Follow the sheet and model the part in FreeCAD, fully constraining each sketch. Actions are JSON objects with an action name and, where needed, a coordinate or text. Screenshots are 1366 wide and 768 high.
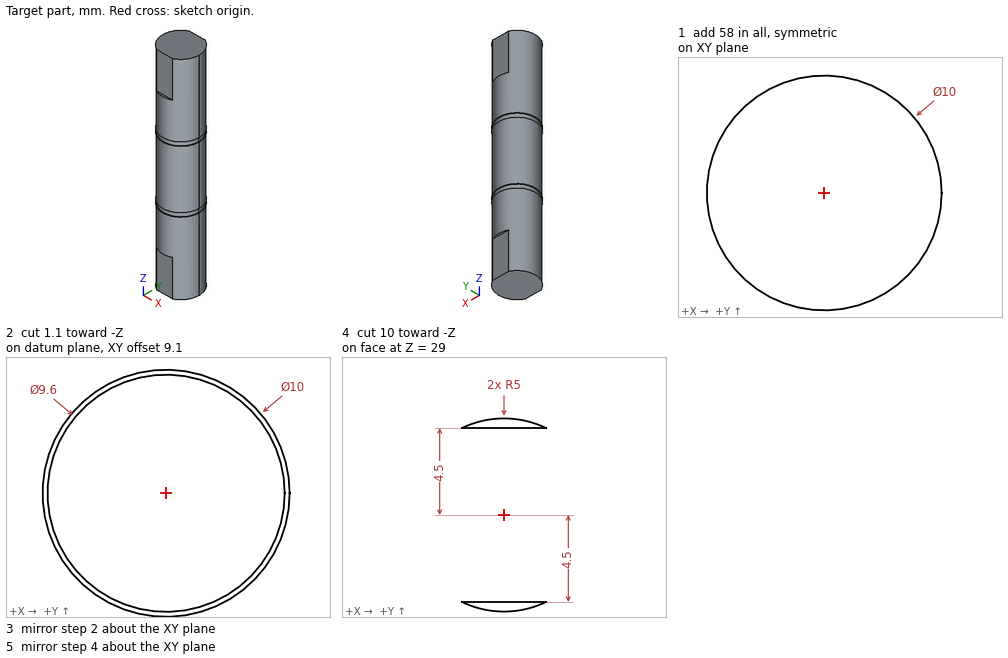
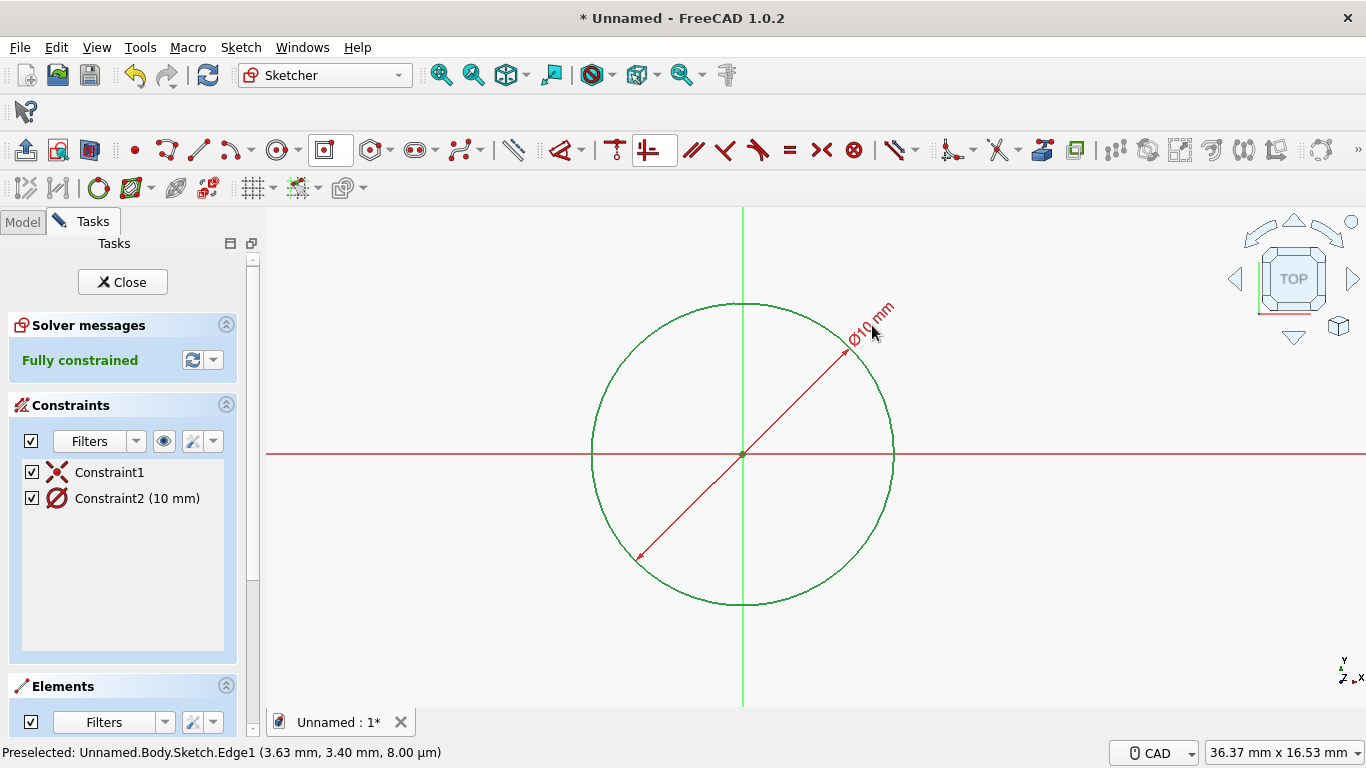
{"action": "left_click", "coordinate": [123, 282]}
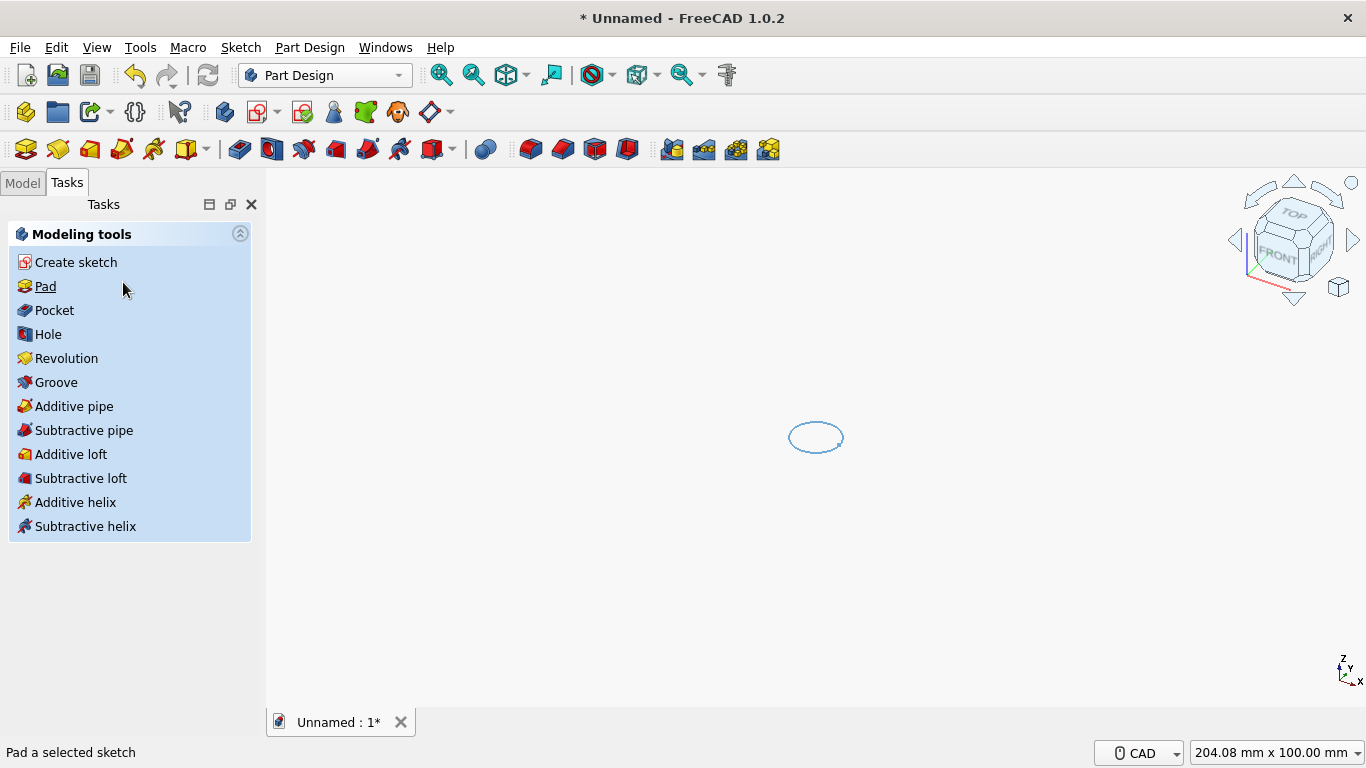
{"action": "left_click", "coordinate": [26, 150]}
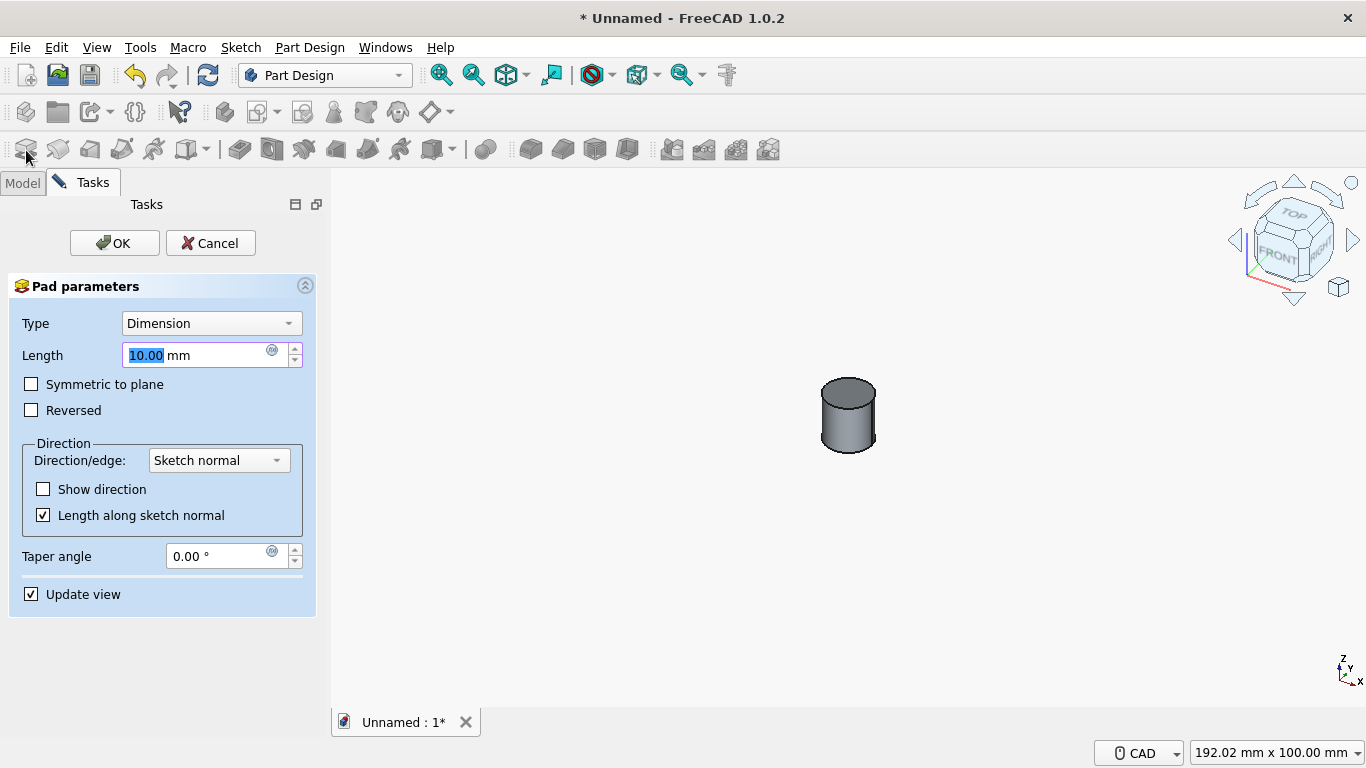
{"action": "type", "text": "58"}
{"action": "key", "text": "Tab"}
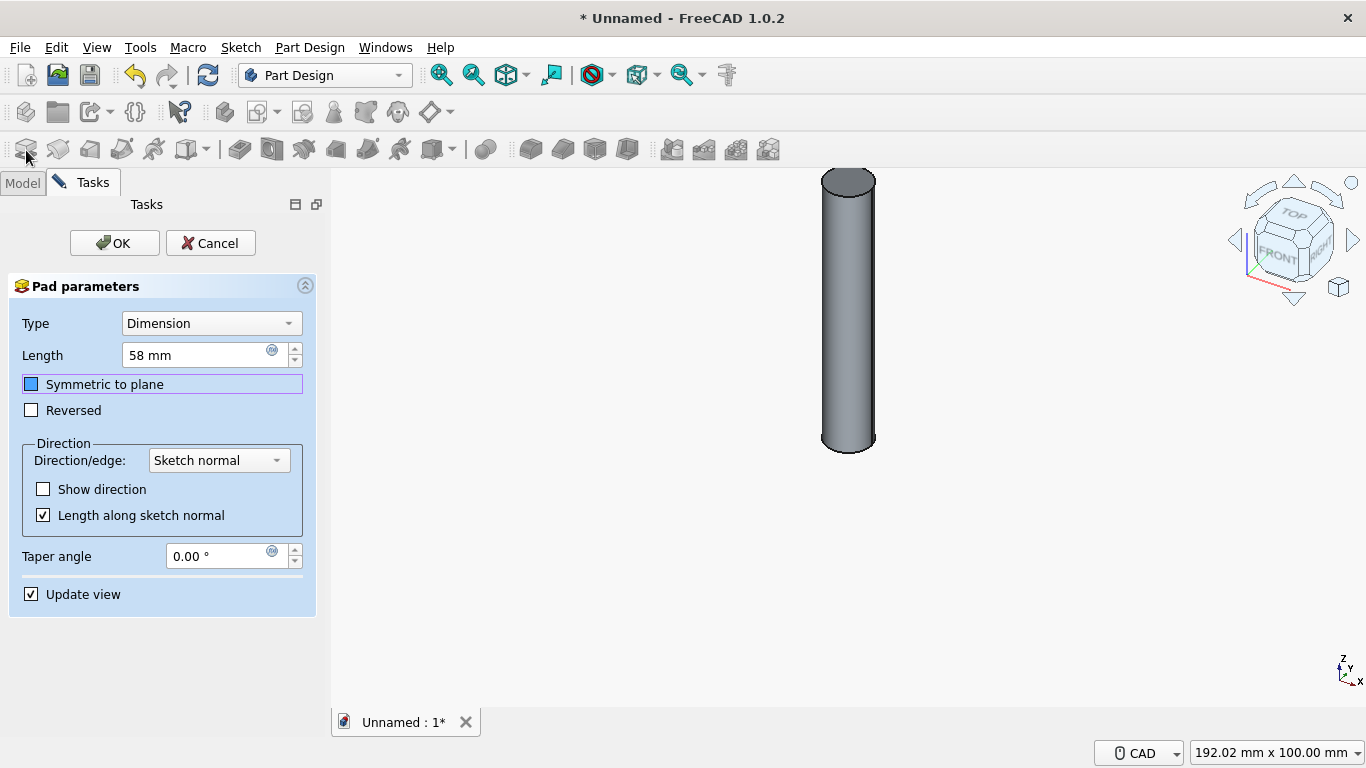
{"action": "left_click", "coordinate": [30, 384]}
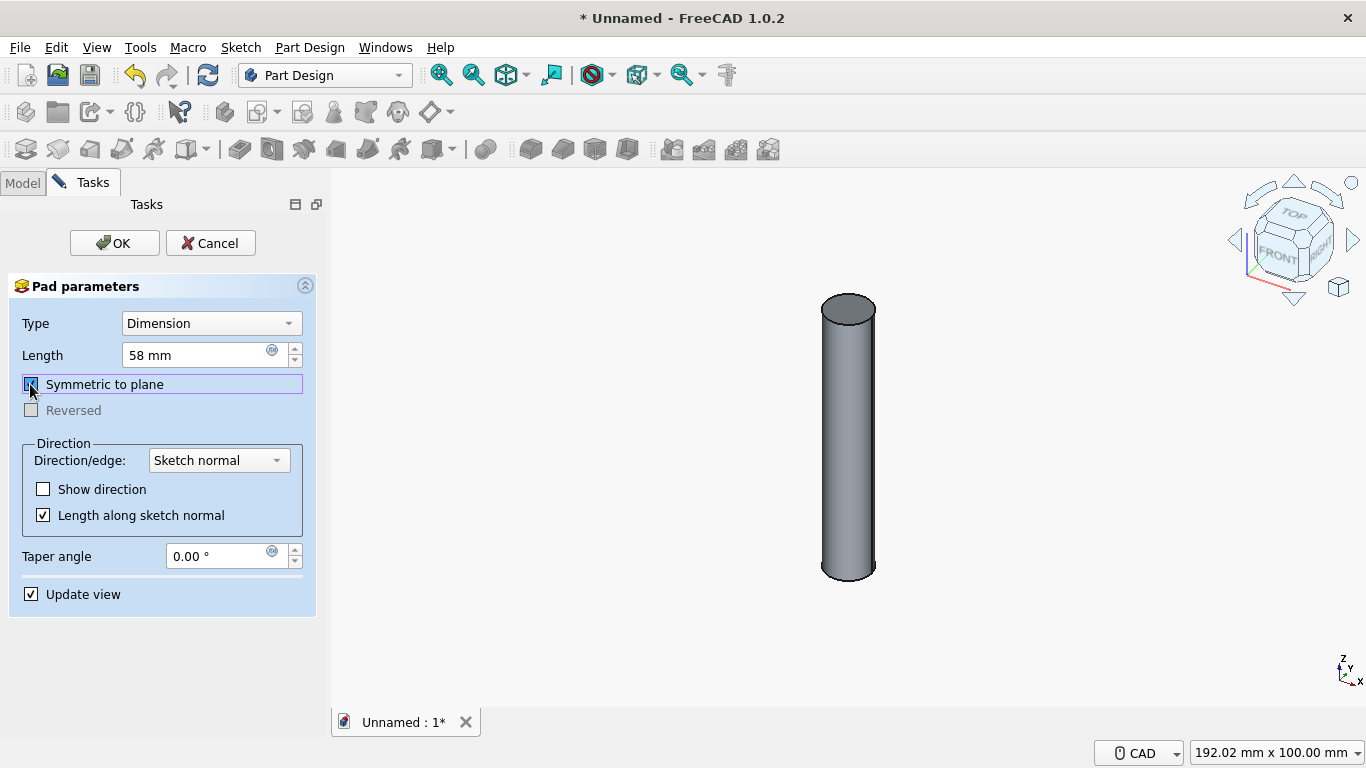
{"action": "left_click", "coordinate": [115, 243]}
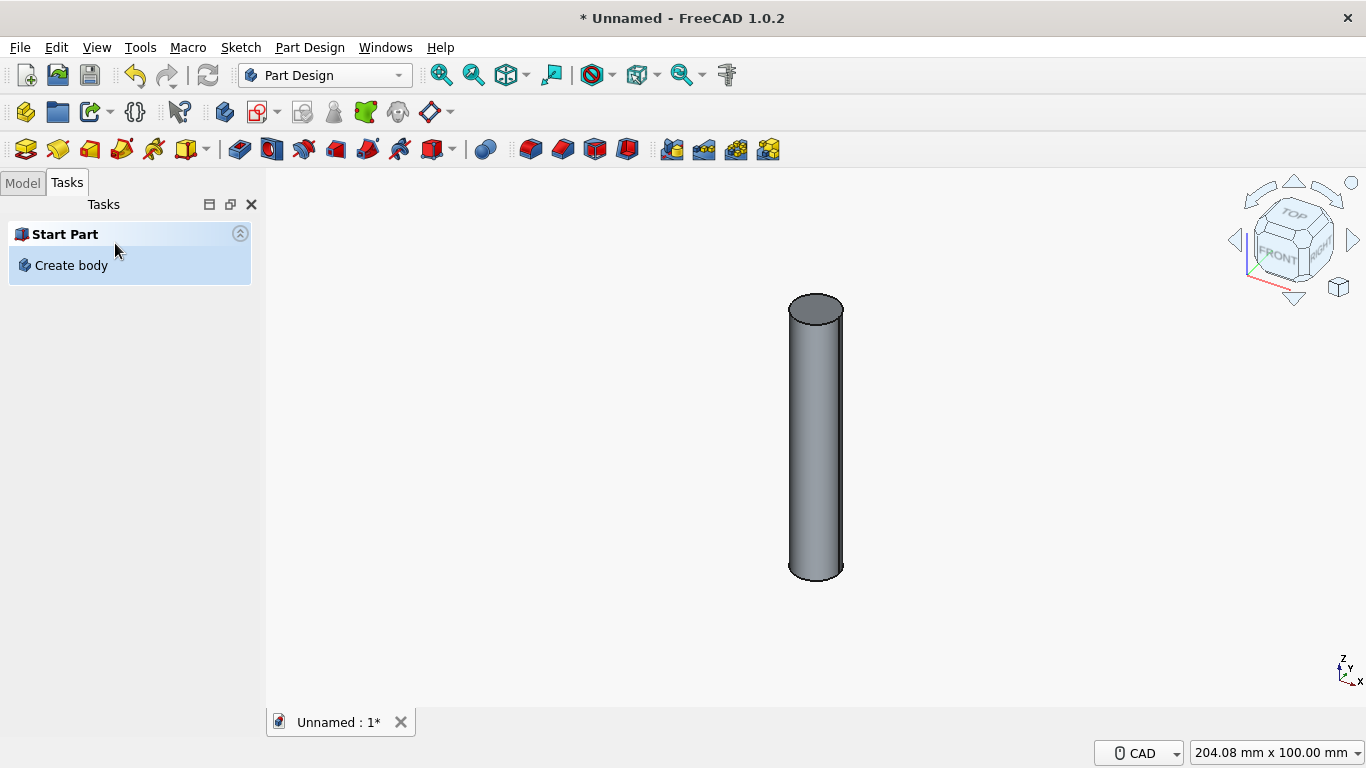
{"action": "left_click", "coordinate": [23, 182]}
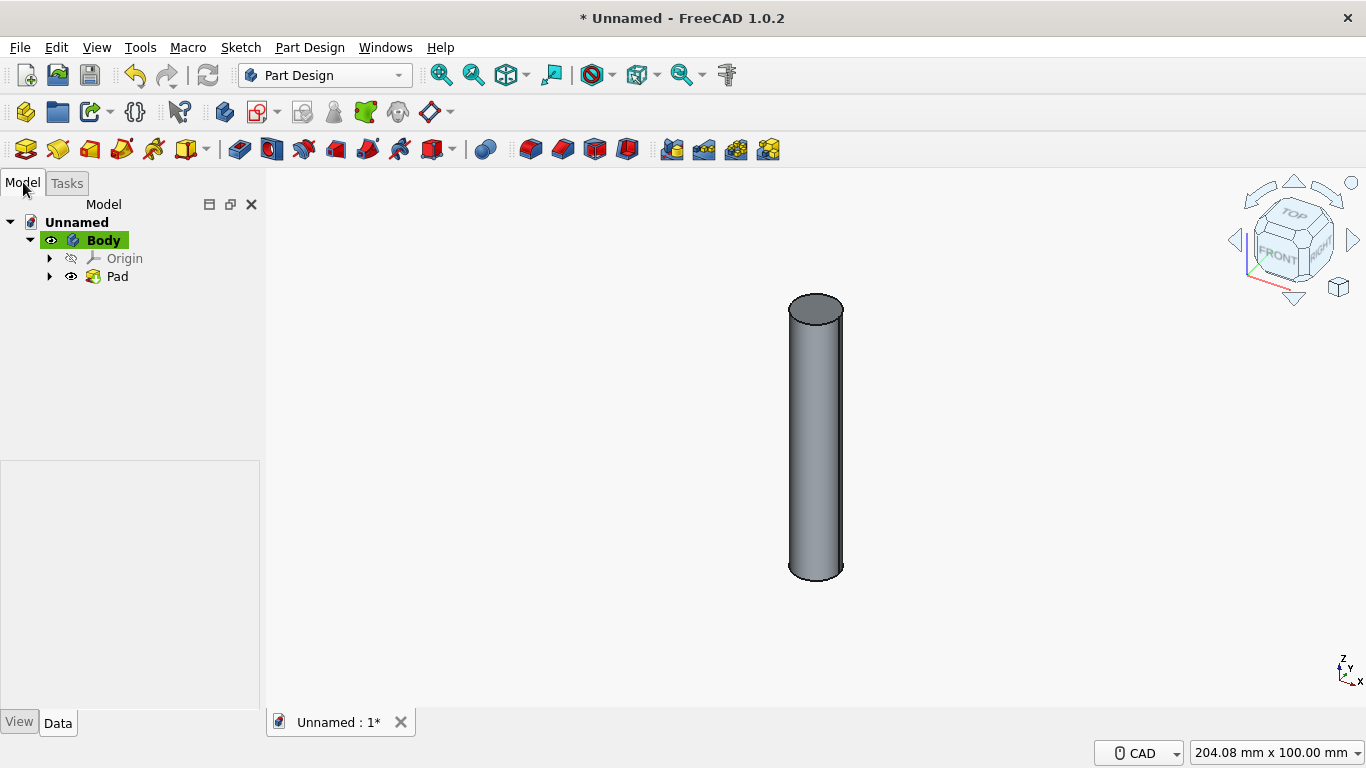
{"action": "left_click", "coordinate": [50, 258]}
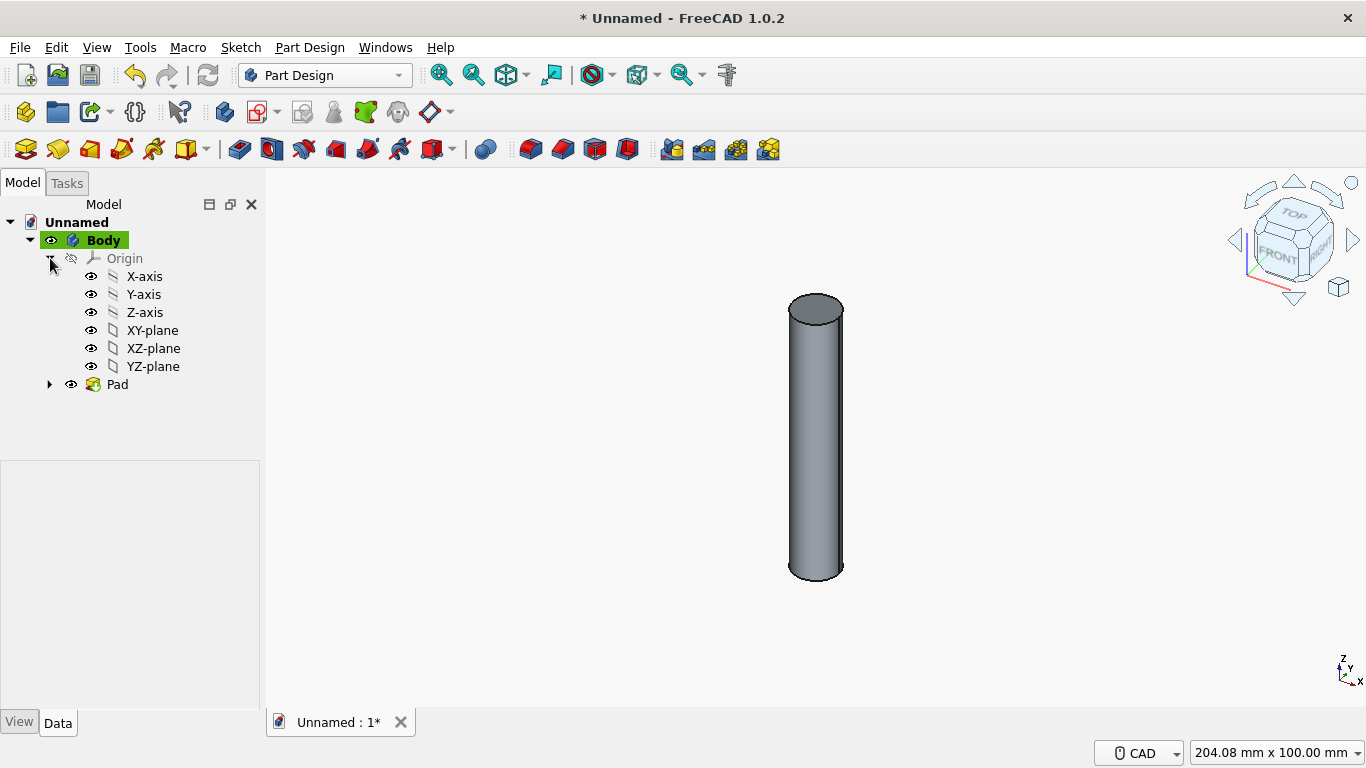
{"action": "left_click", "coordinate": [136, 330]}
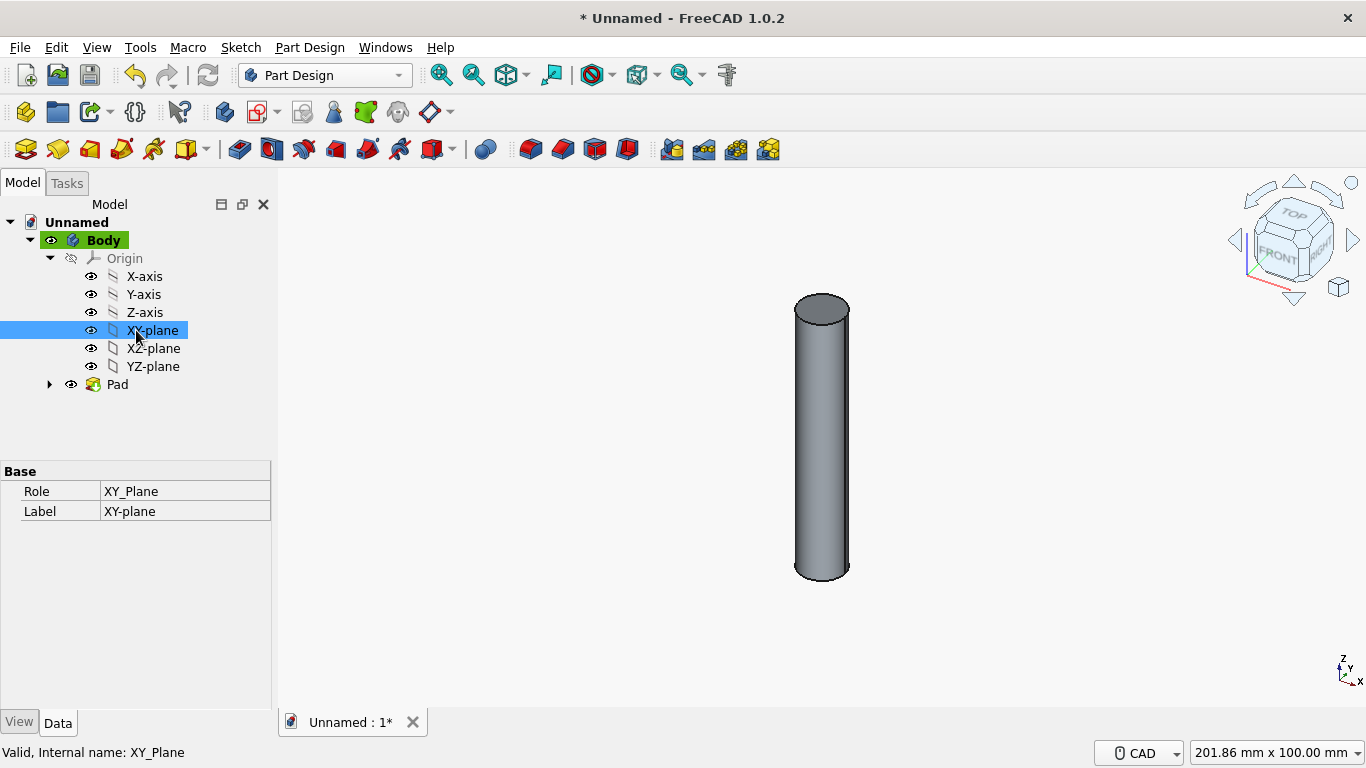
{"action": "left_click", "coordinate": [430, 112]}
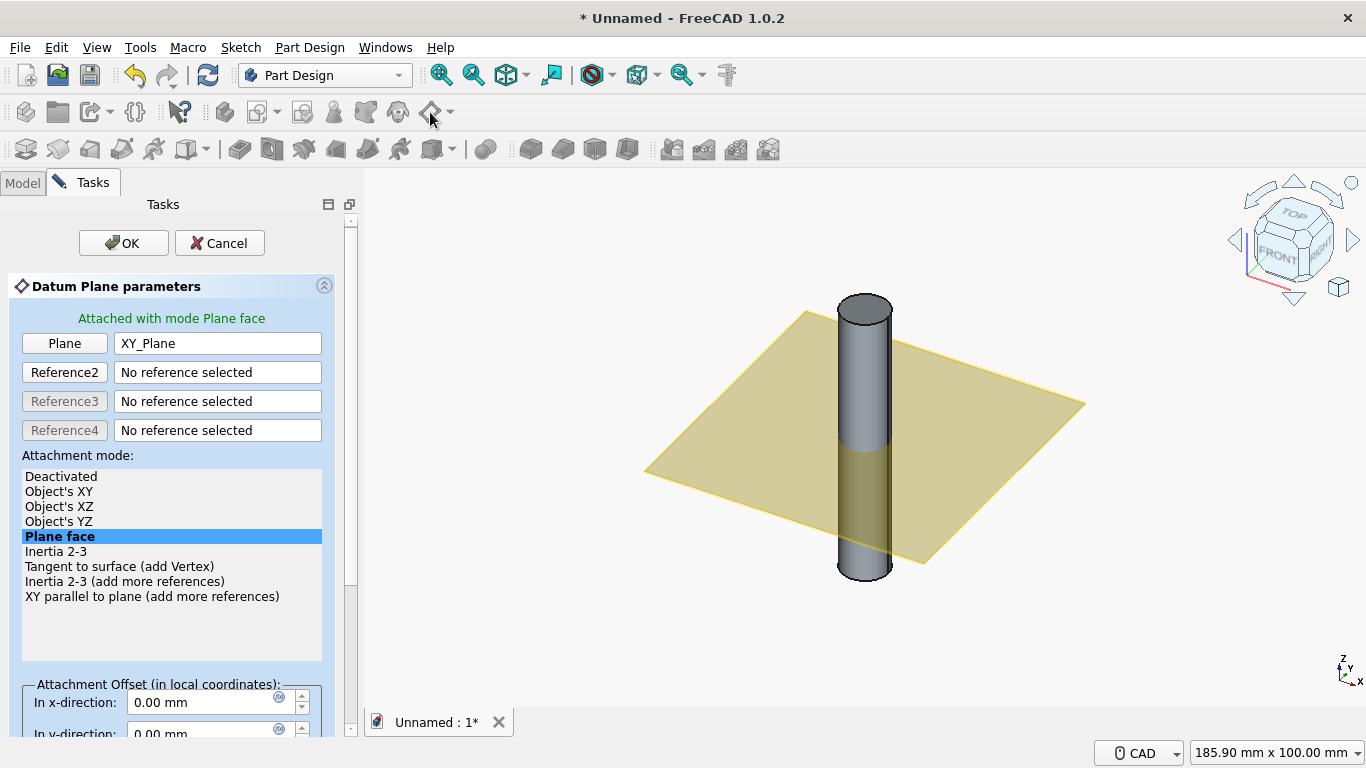
{"action": "scroll", "coordinate": [351, 475], "scroll_direction": "down", "scroll_amount": 2}